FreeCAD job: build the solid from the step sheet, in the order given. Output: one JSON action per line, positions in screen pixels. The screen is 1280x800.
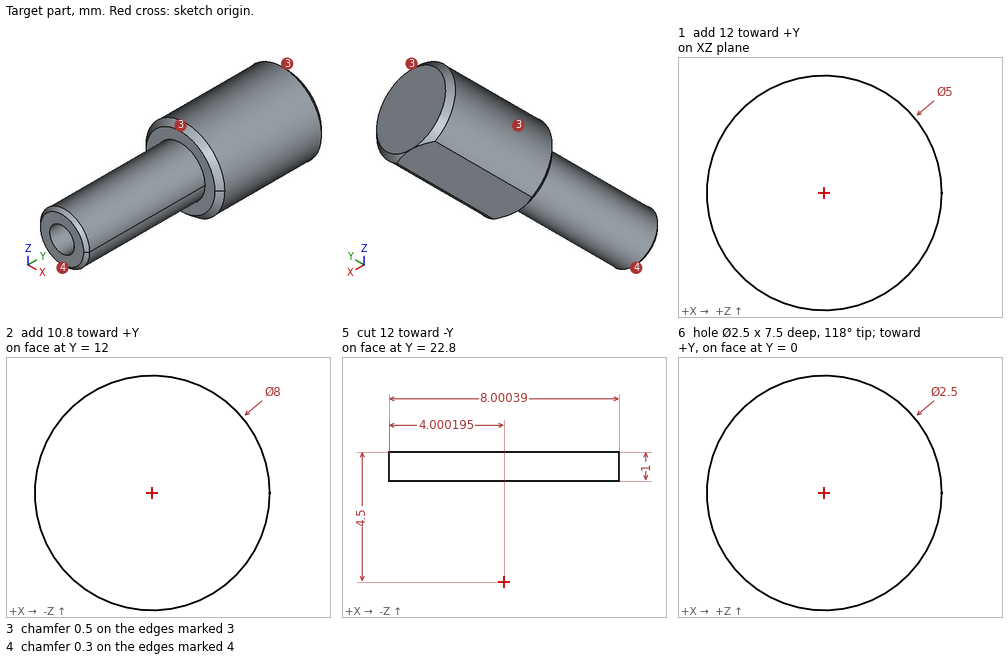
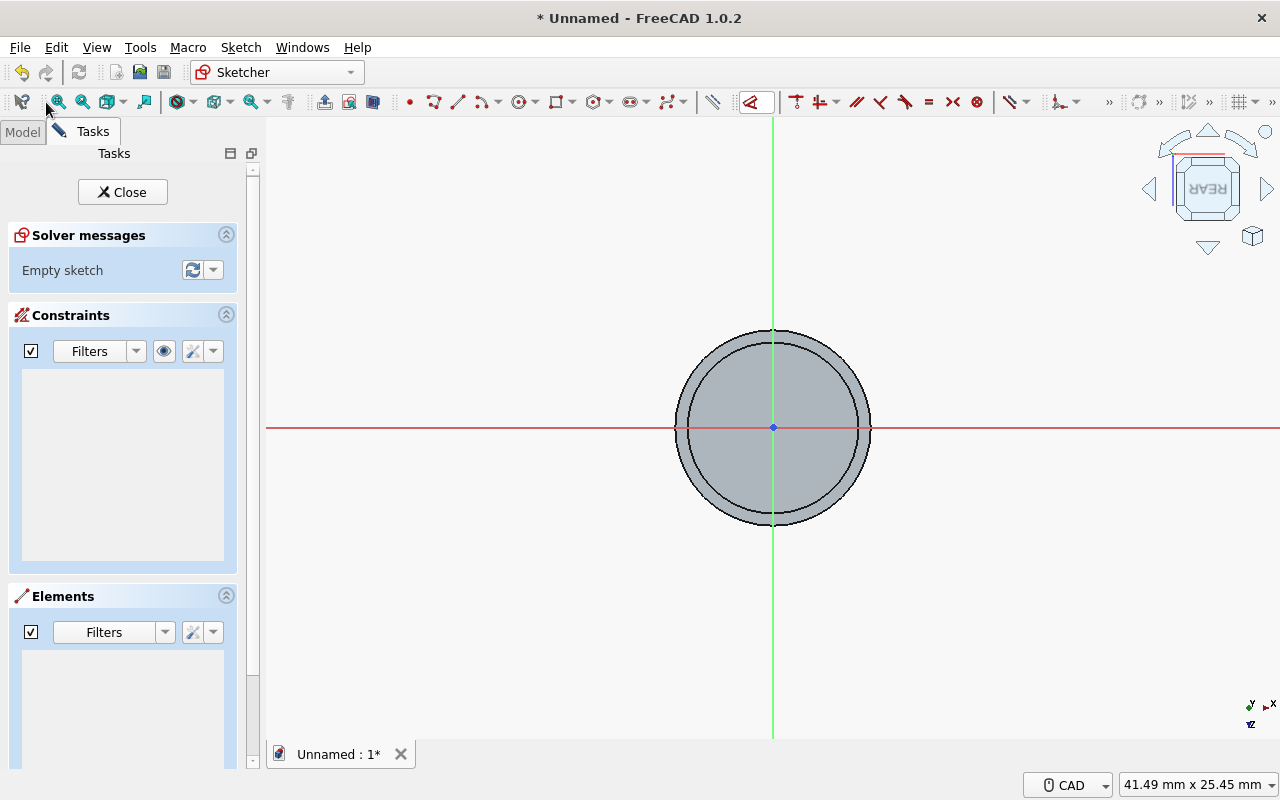
{"action": "scroll", "coordinate": [813, 341], "scroll_direction": "up", "scroll_amount": 5}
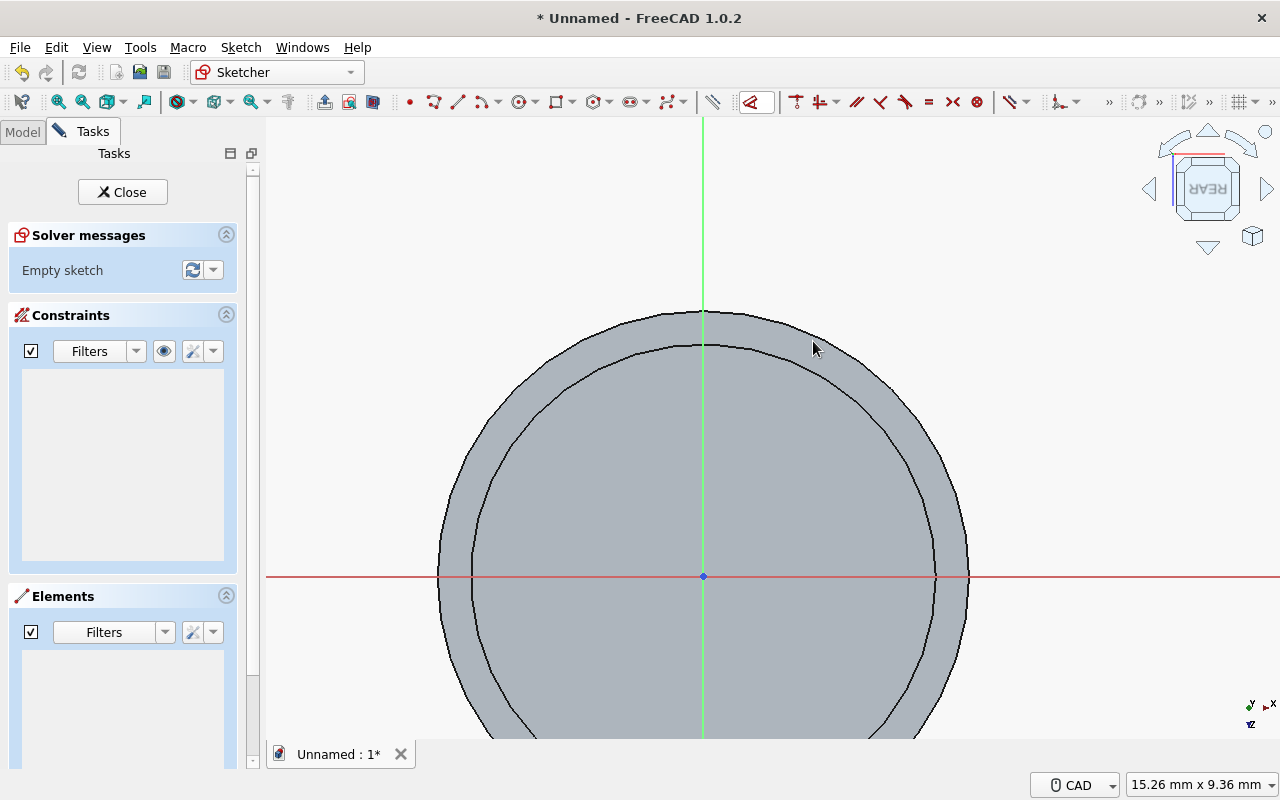
{"action": "left_click", "coordinate": [556, 102]}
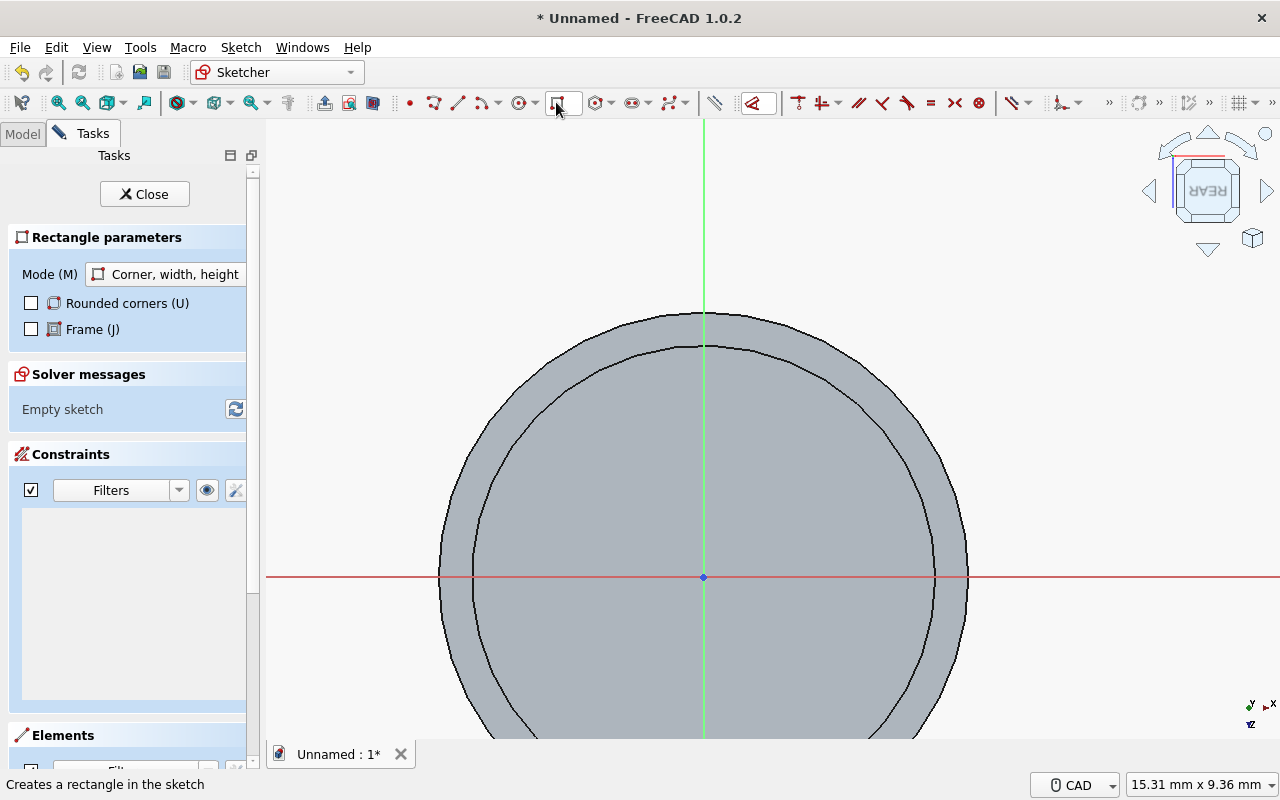
{"action": "left_click", "coordinate": [439, 279]}
{"action": "mouse_move", "coordinate": [968, 346]}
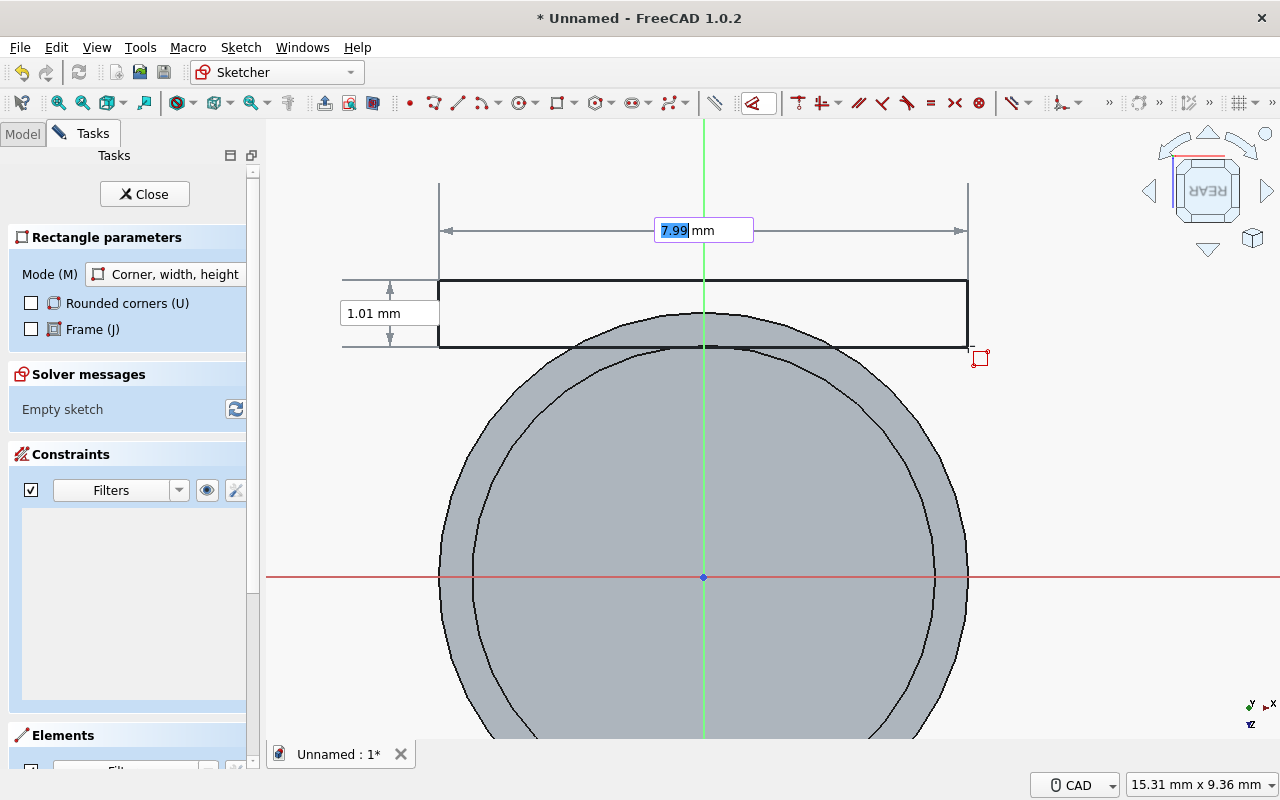
{"action": "type", "text": "8.00039"}
{"action": "key", "text": "Tab"}
{"action": "type", "text": "1"}
{"action": "key", "text": "Return"}
{"action": "key", "text": "Escape"}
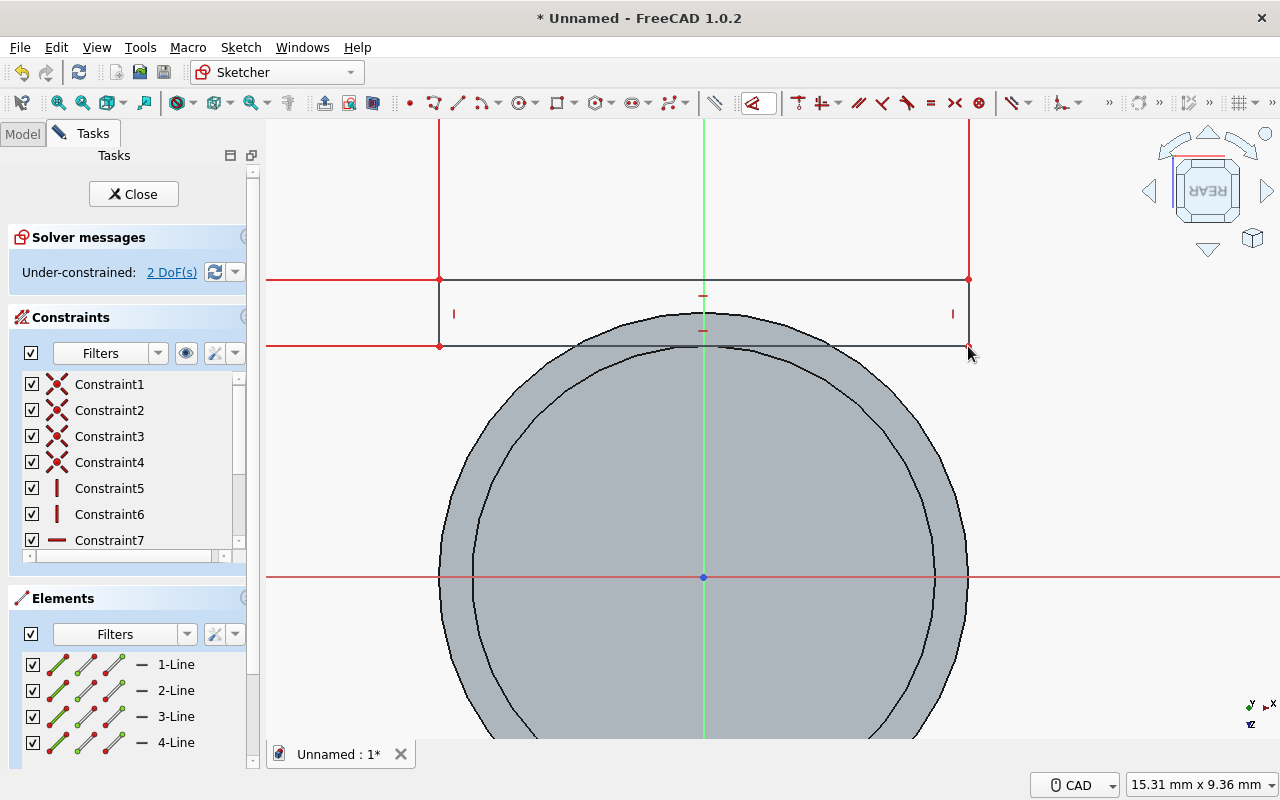
{"action": "left_click", "coordinate": [439, 280]}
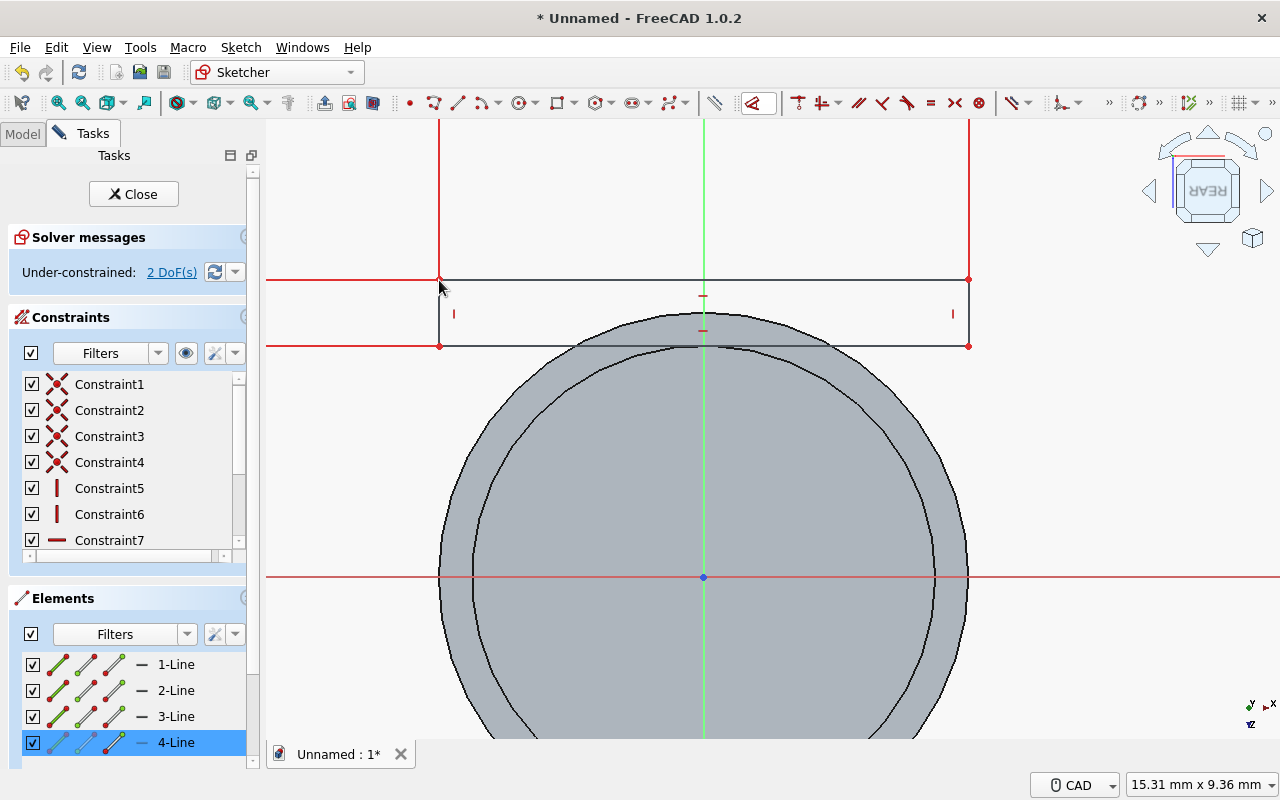
{"action": "left_click", "coordinate": [770, 104]}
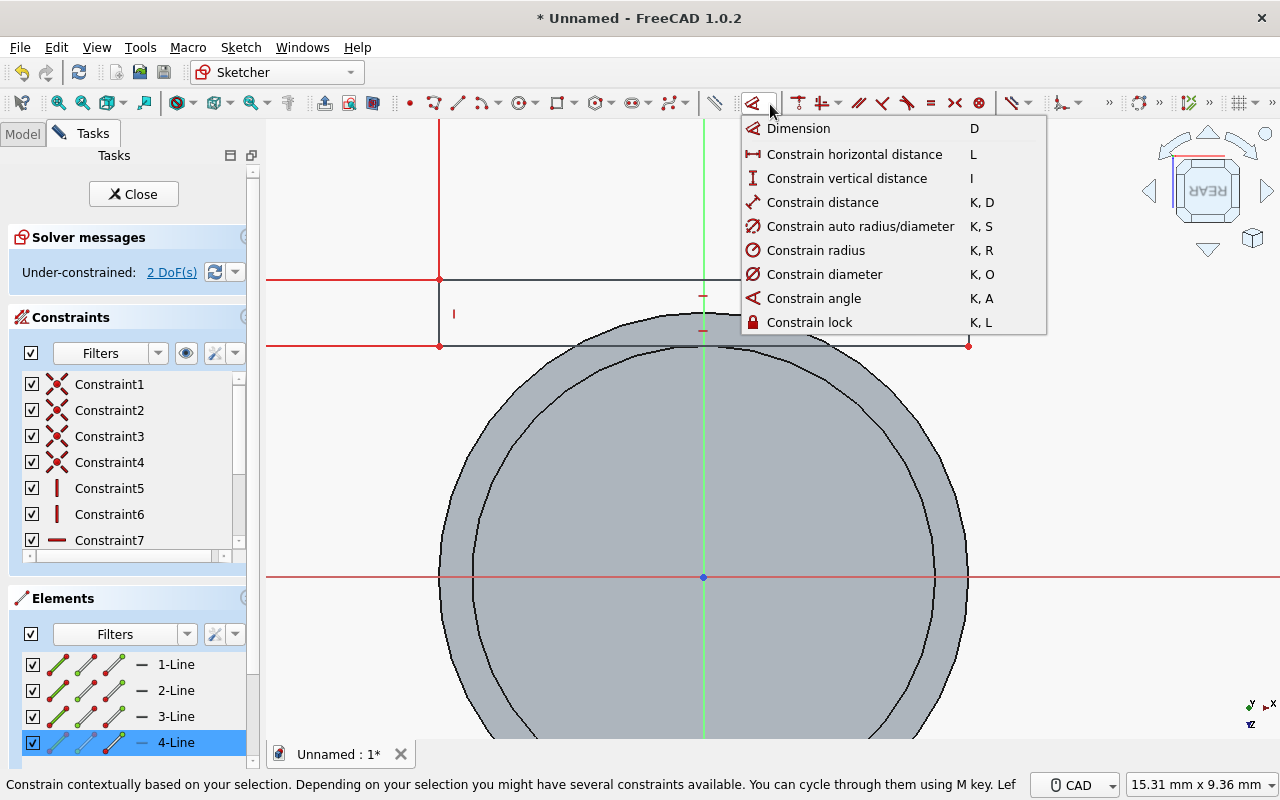
{"action": "left_click", "coordinate": [894, 178]}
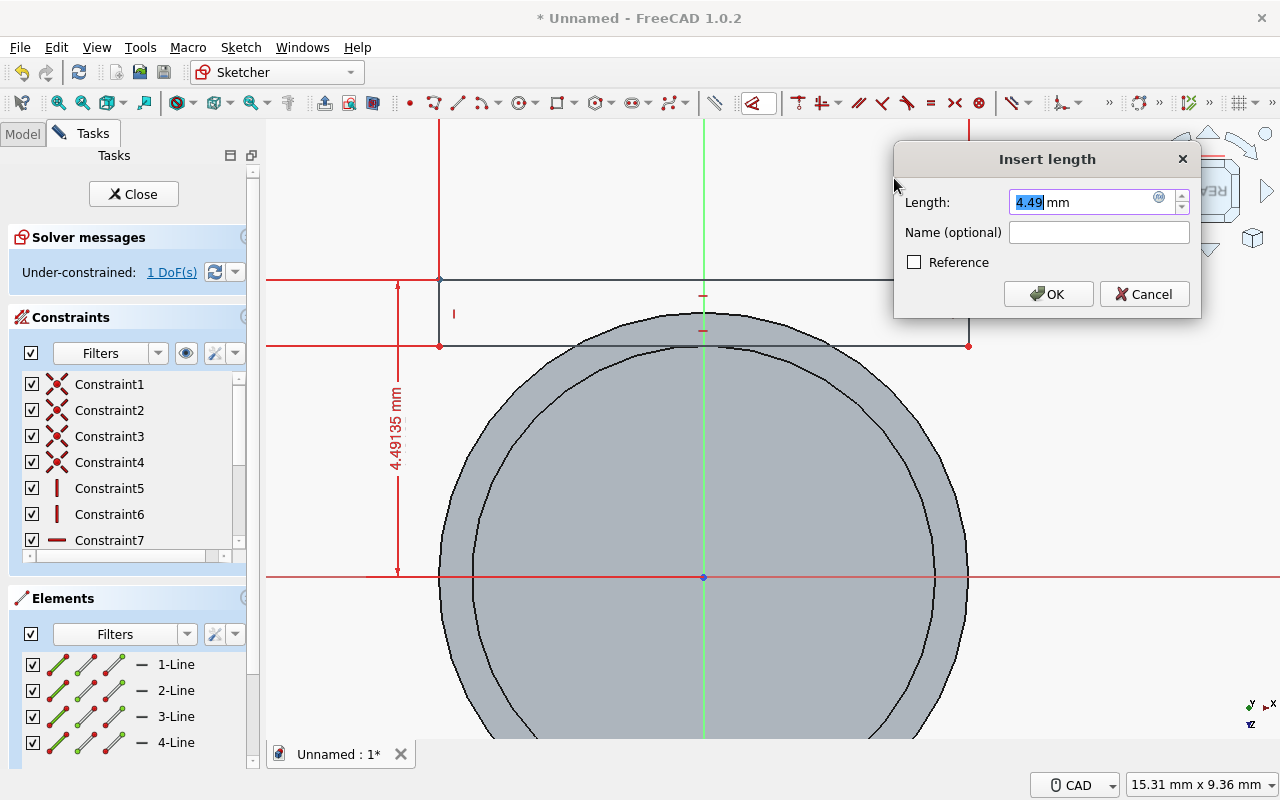
{"action": "type", "text": "4.5"}
{"action": "key", "text": "Return"}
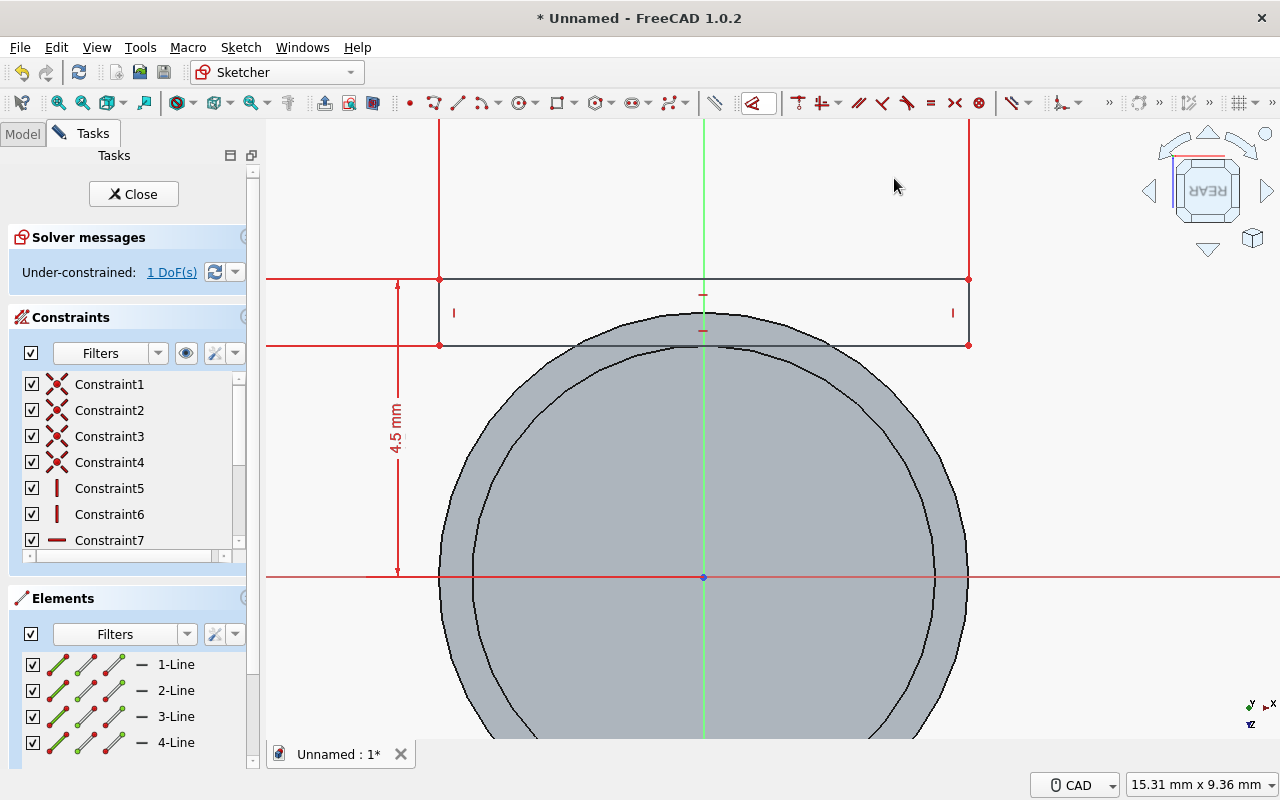
{"action": "left_click", "coordinate": [439, 279]}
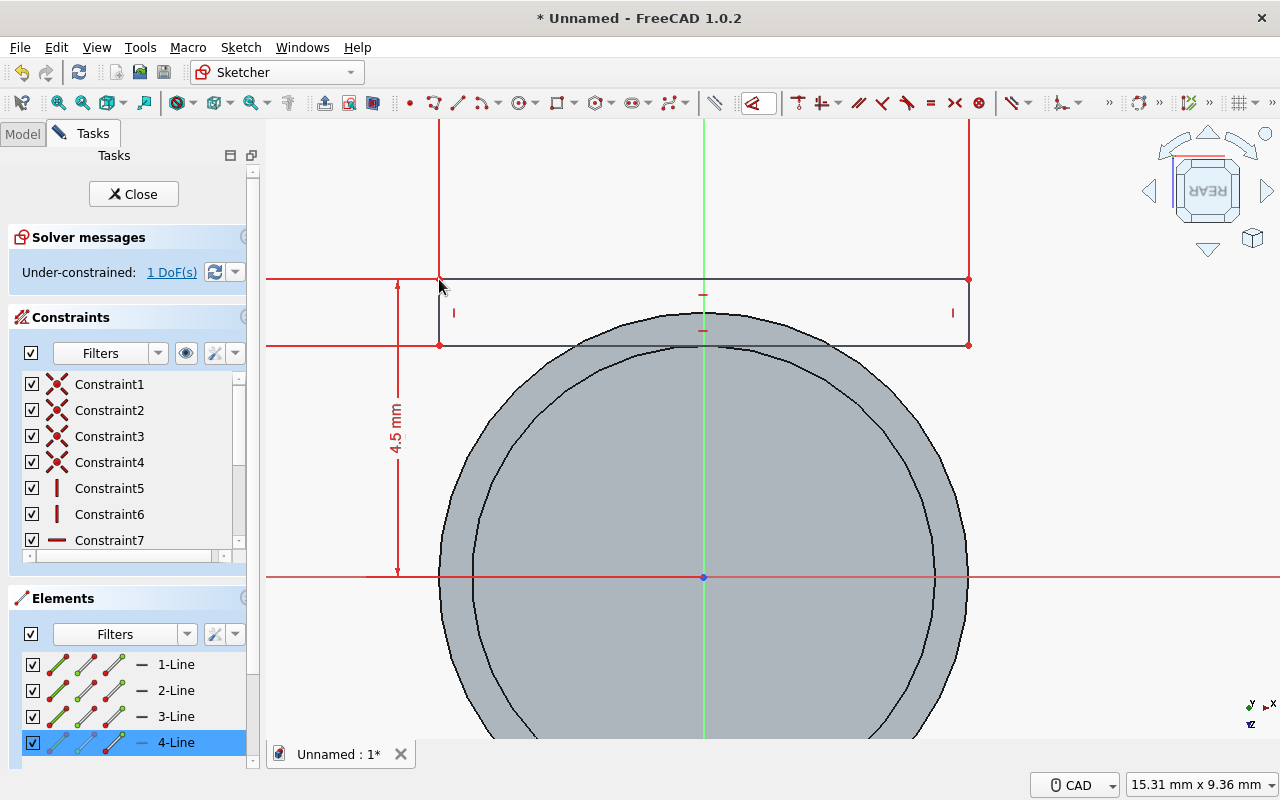
{"action": "key", "text": "l"}